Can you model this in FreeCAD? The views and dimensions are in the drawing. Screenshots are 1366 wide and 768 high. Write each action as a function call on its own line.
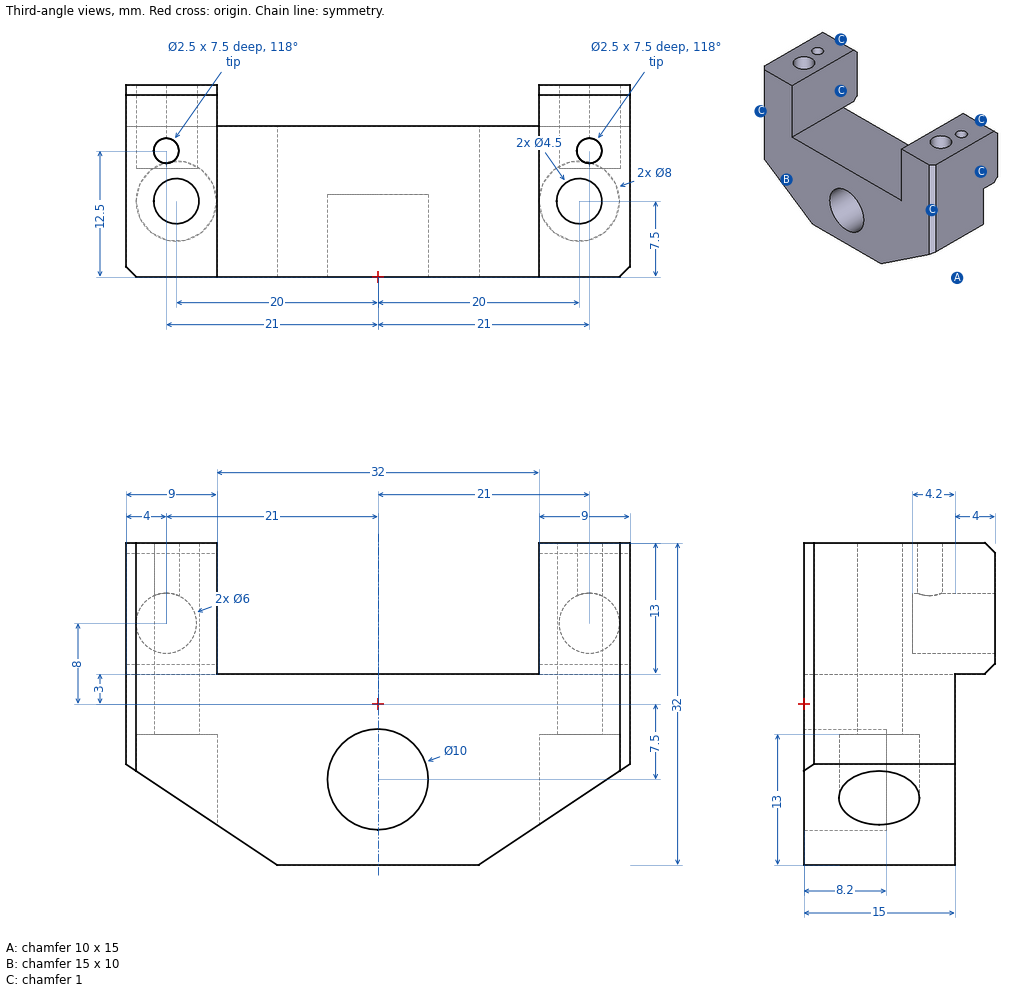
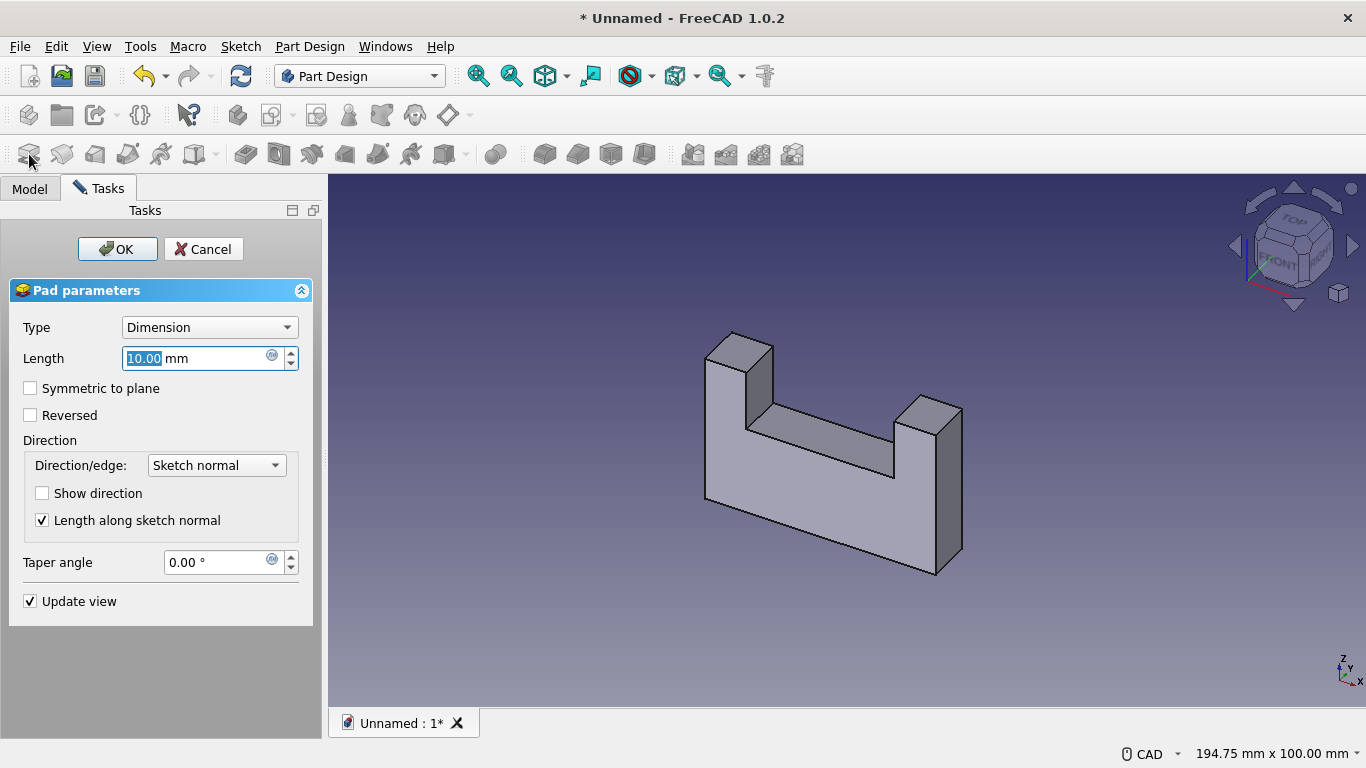
text(15)
key(Tab)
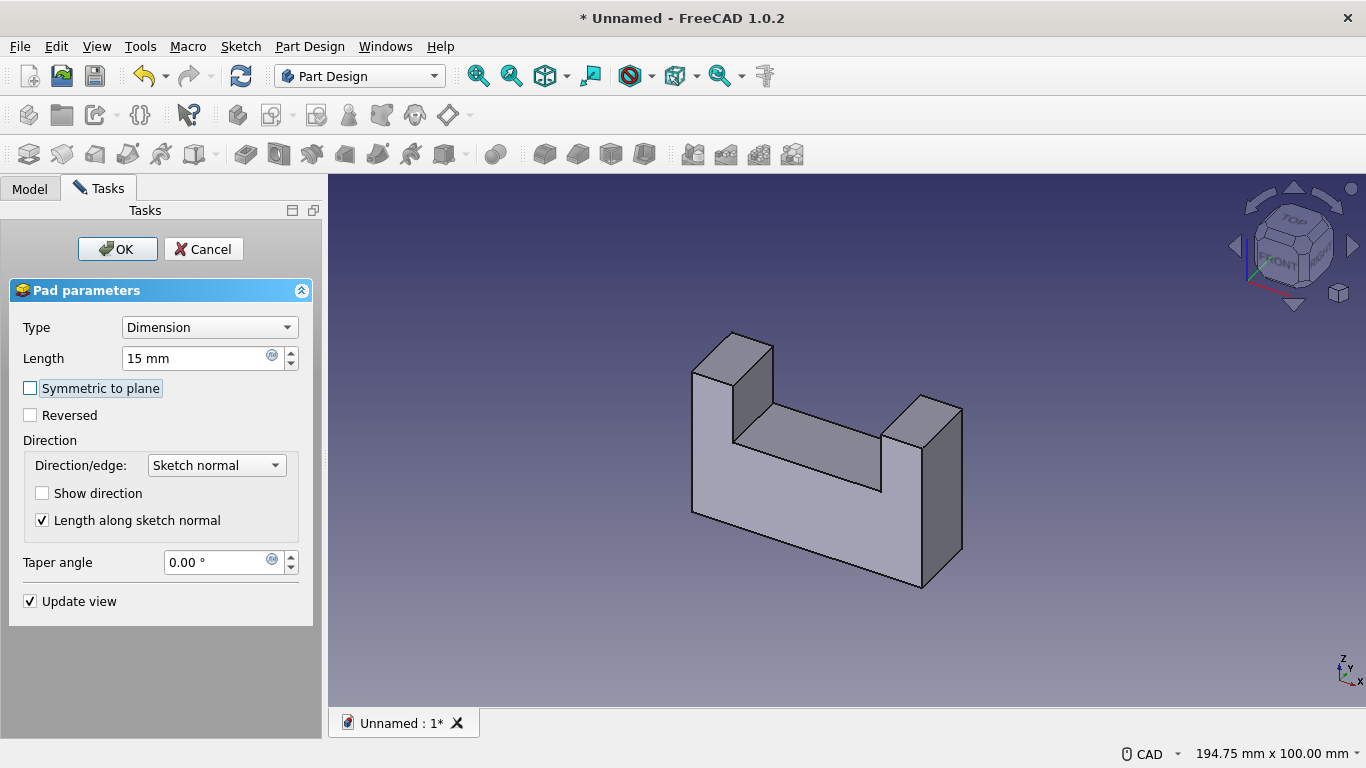
click(31, 415)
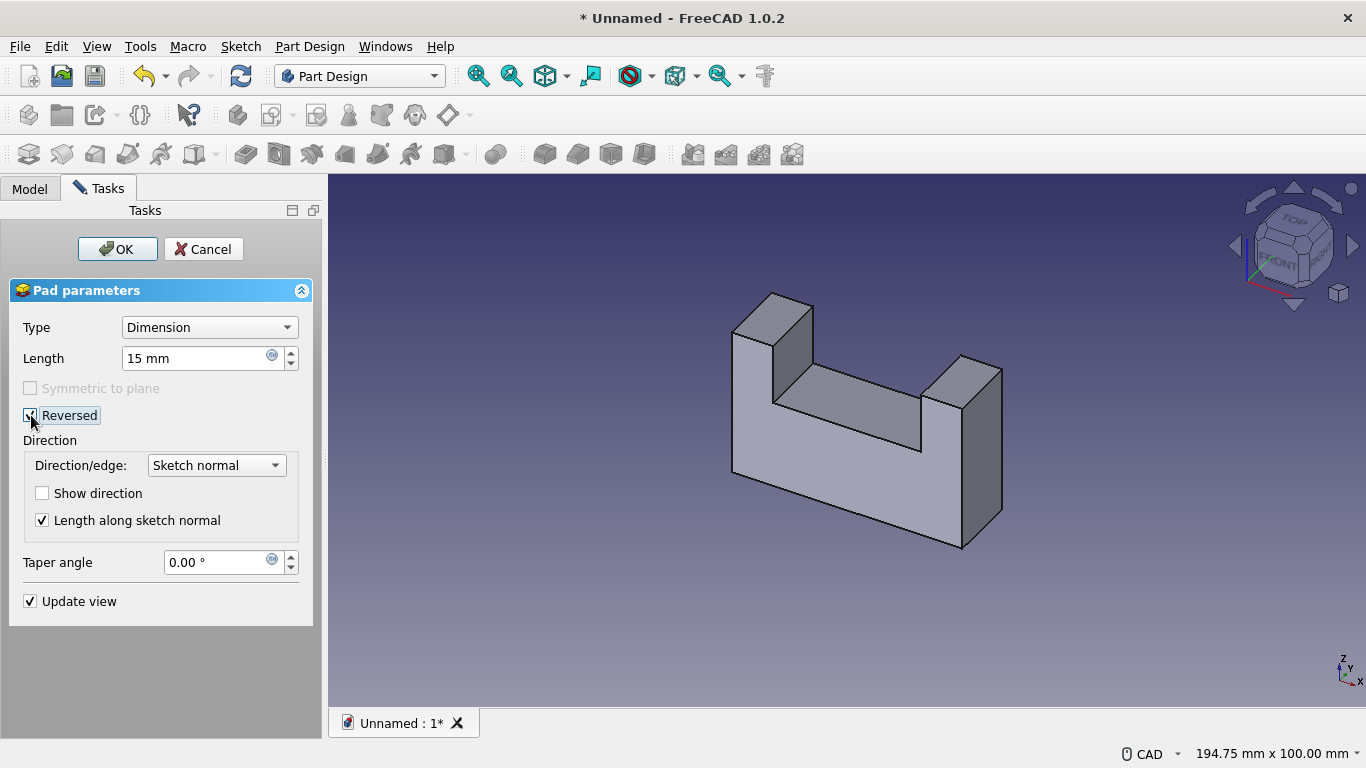
click(118, 249)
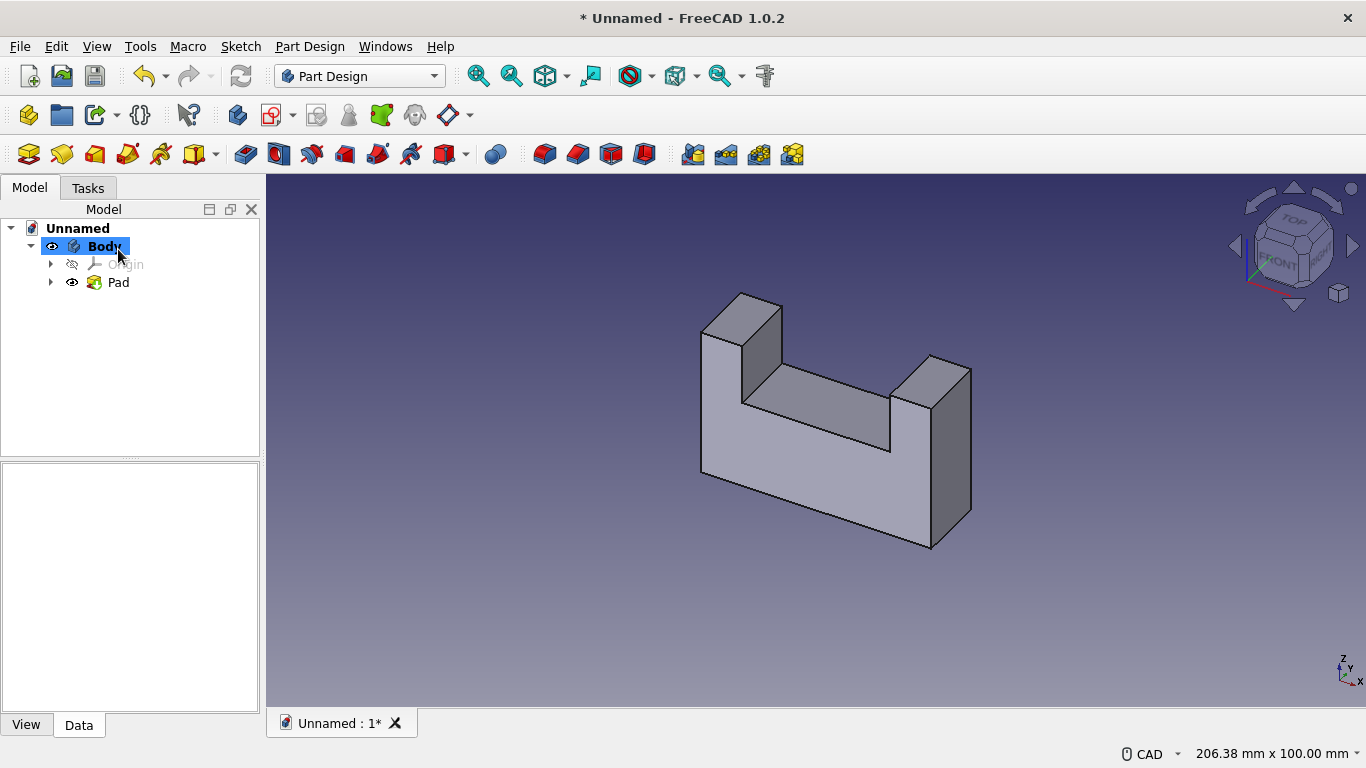
key(0)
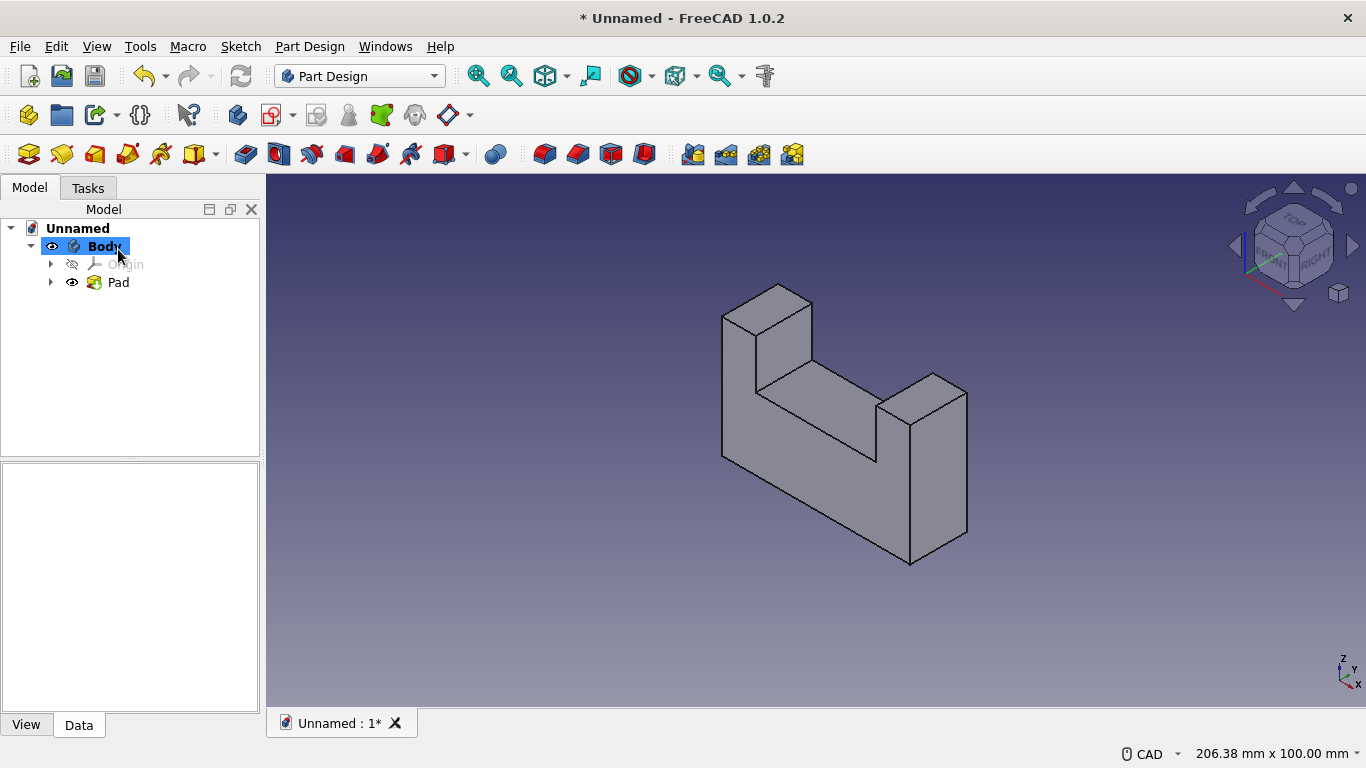
key(2)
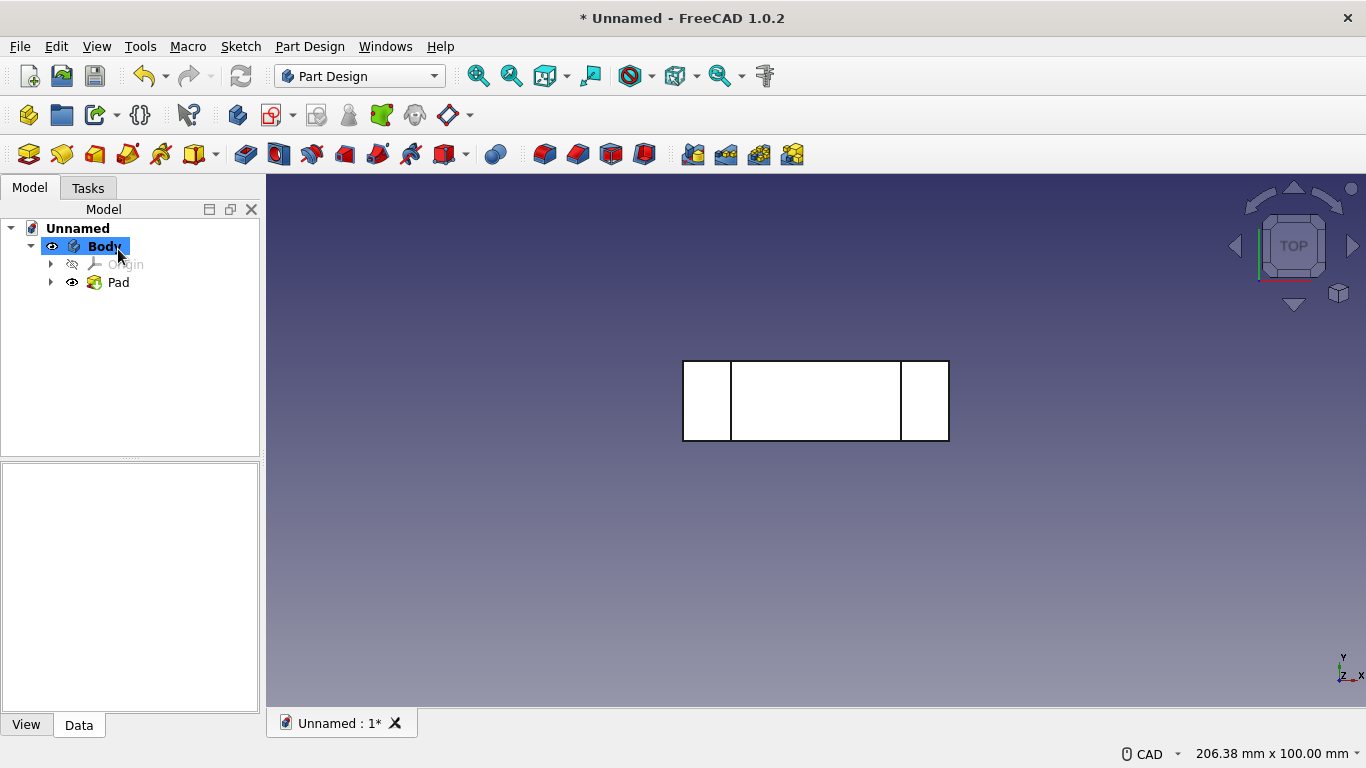
click(479, 76)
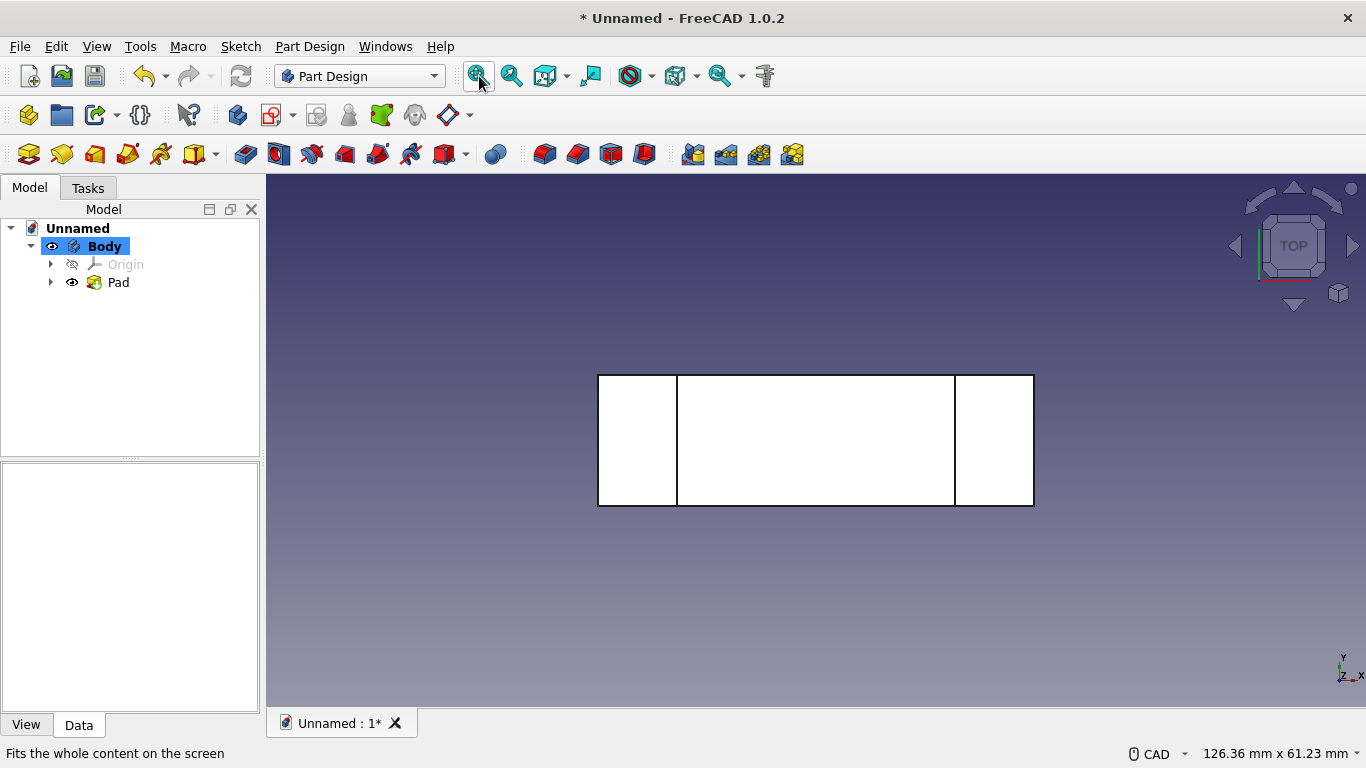
key(1)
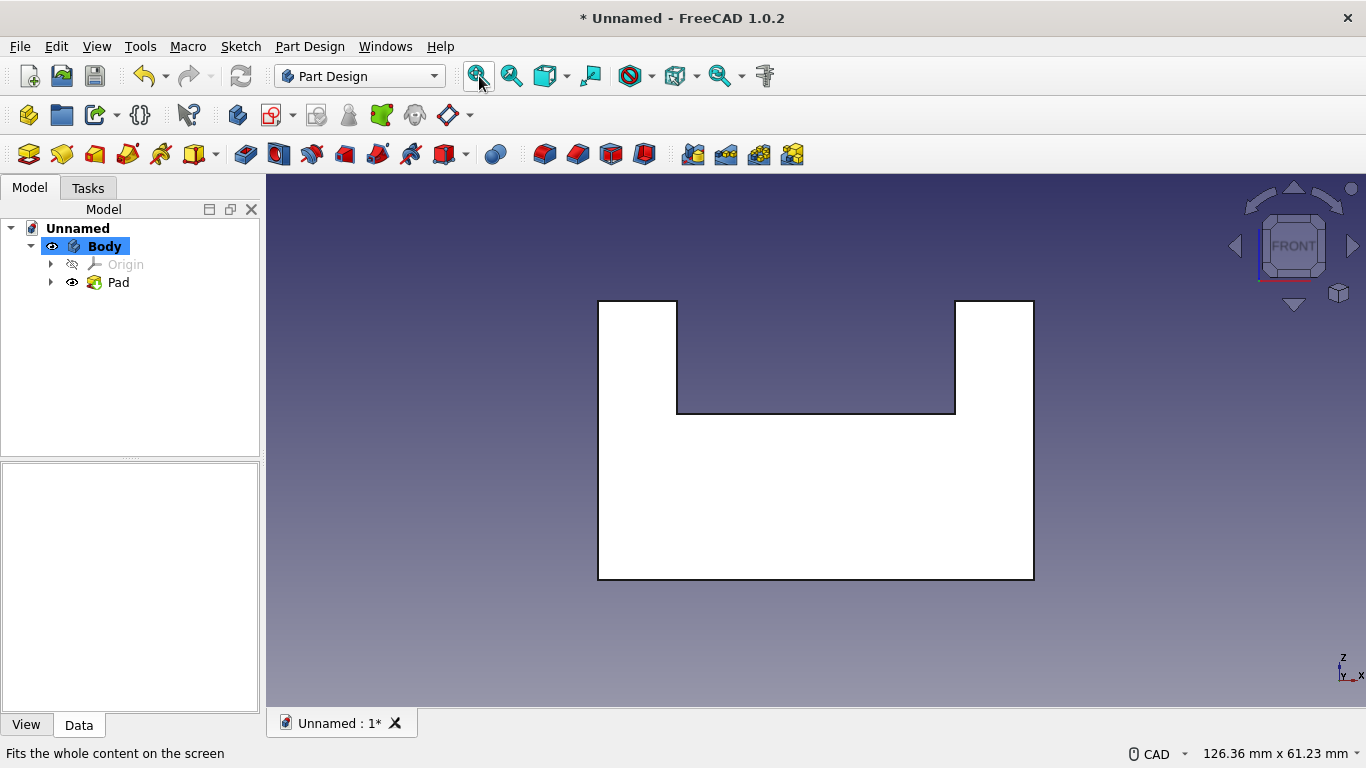
key(3)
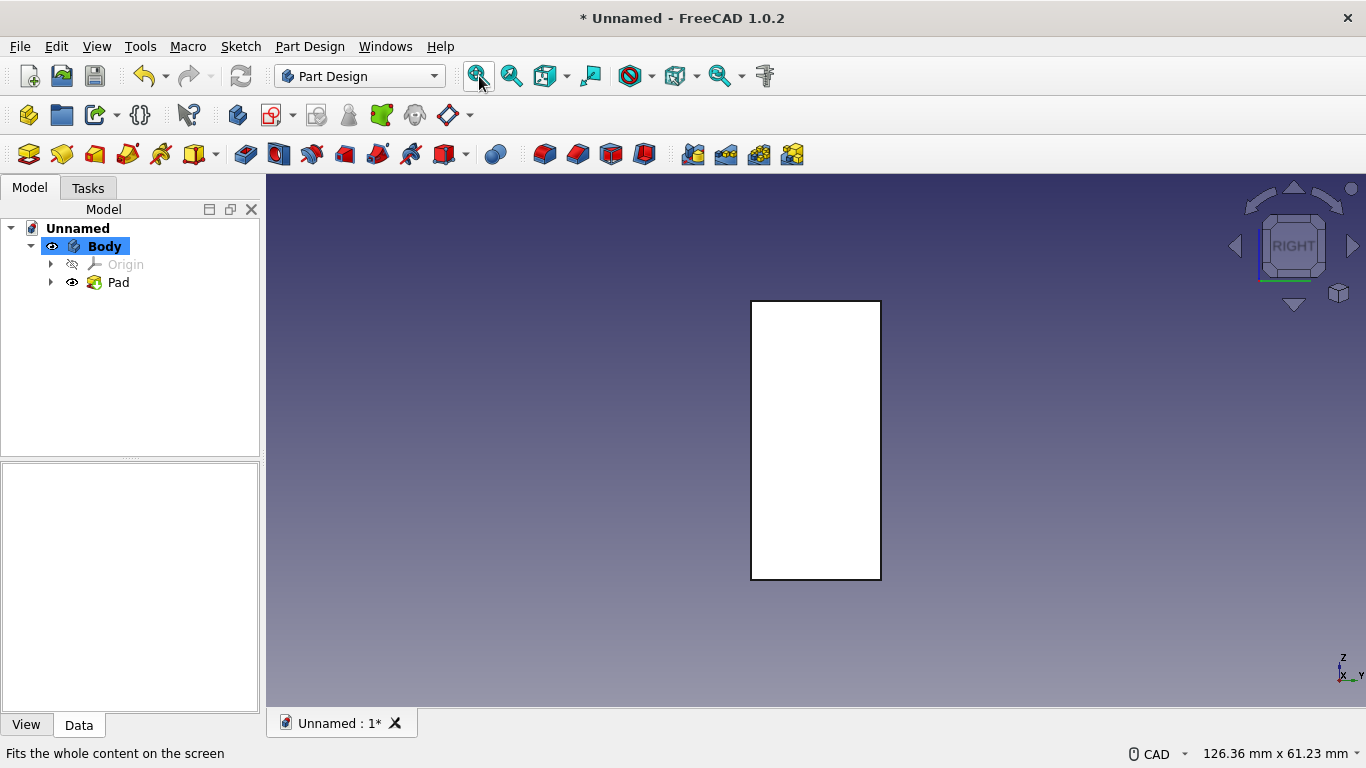
click(816, 579)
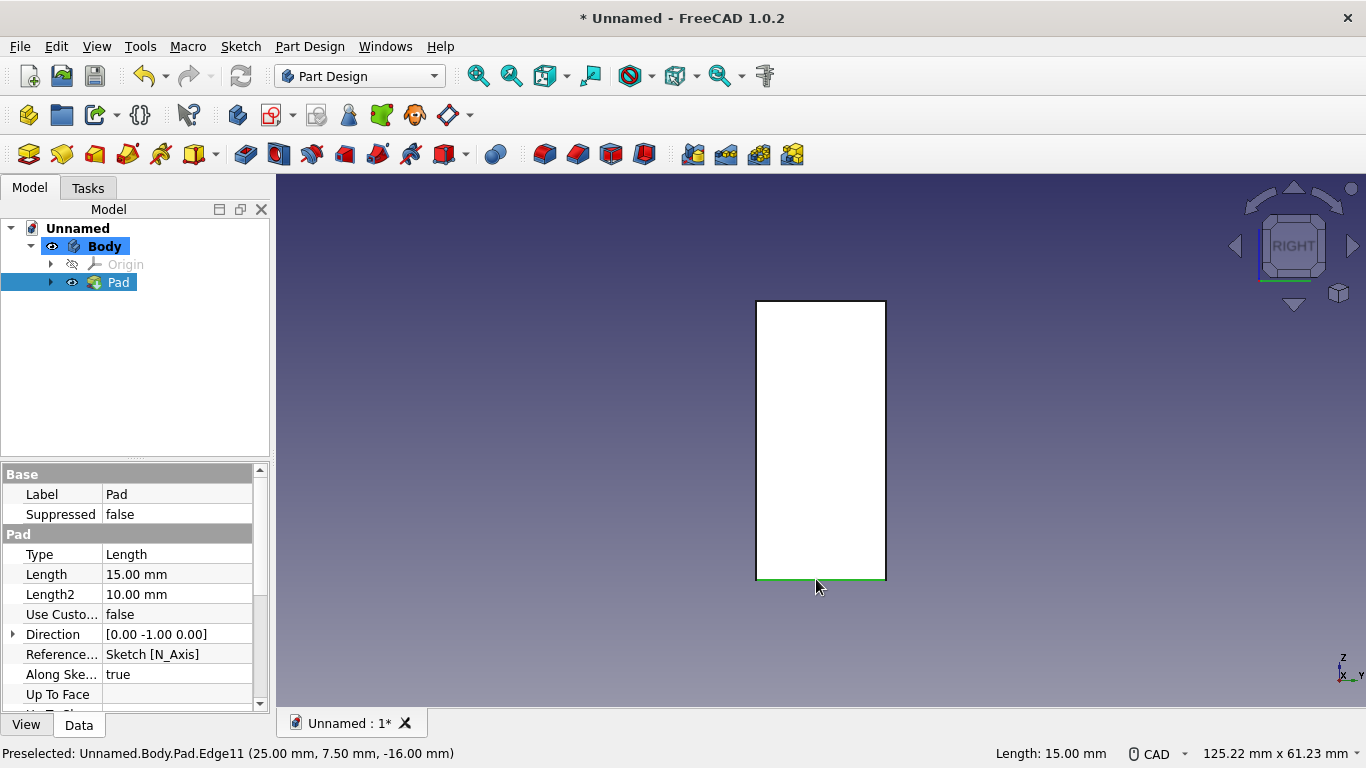
click(578, 154)